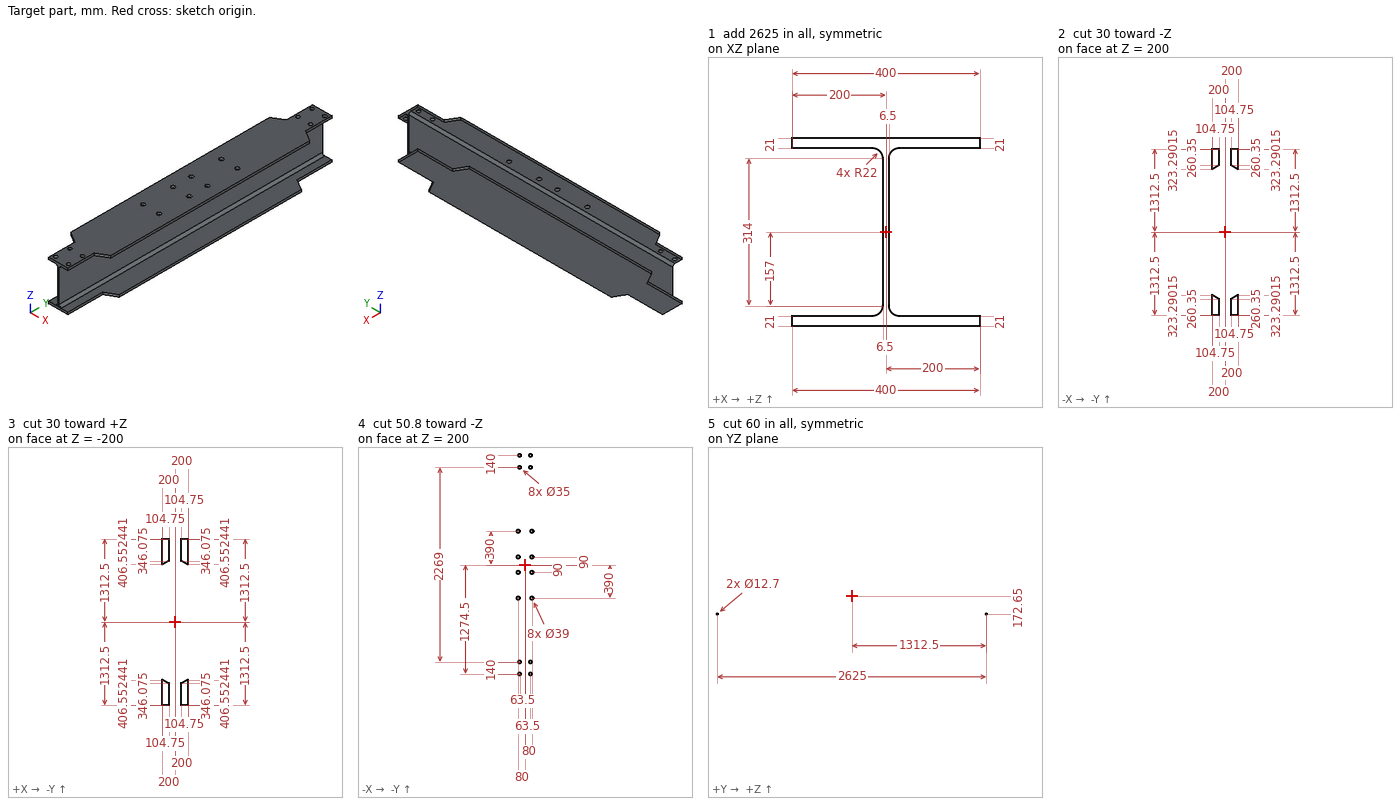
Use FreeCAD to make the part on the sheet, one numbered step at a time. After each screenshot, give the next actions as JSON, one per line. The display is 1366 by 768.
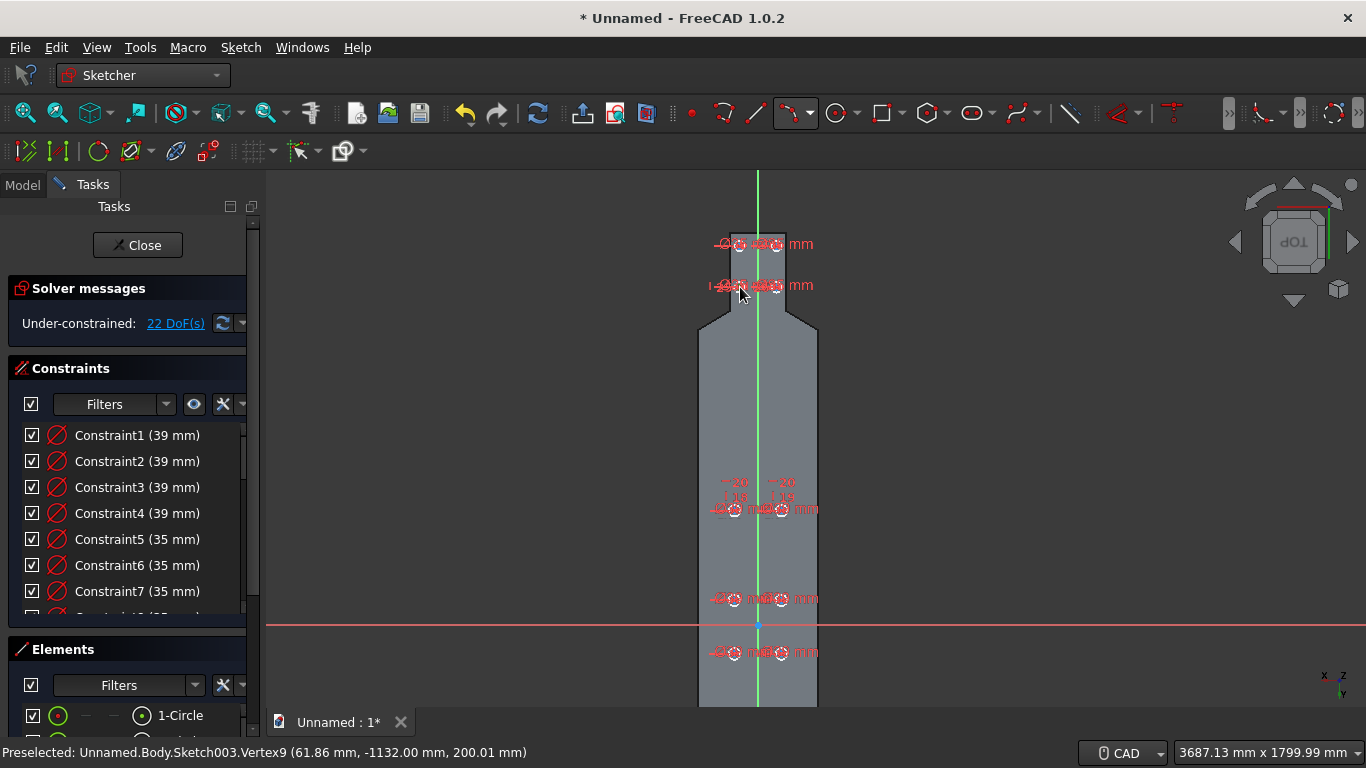
{"action": "left_click", "coordinate": [777, 287]}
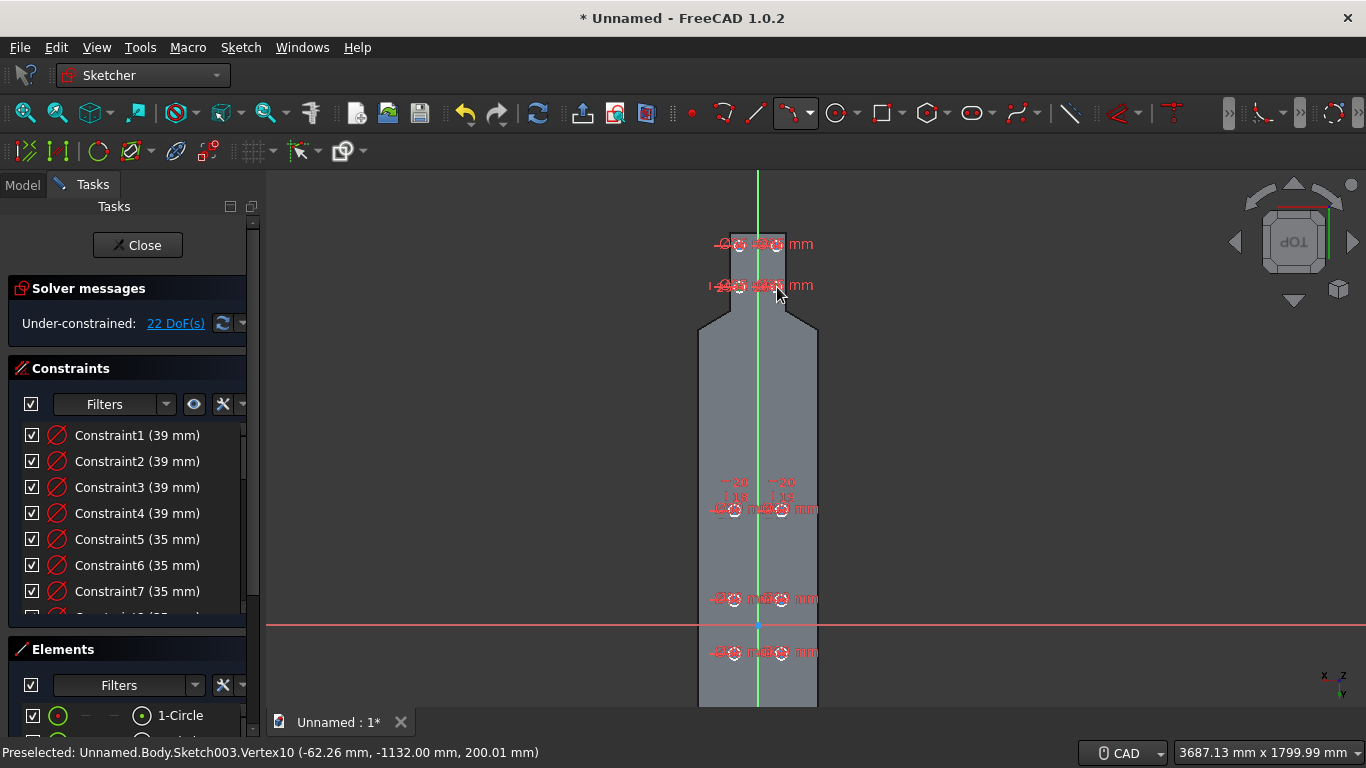
{"action": "key", "text": "h"}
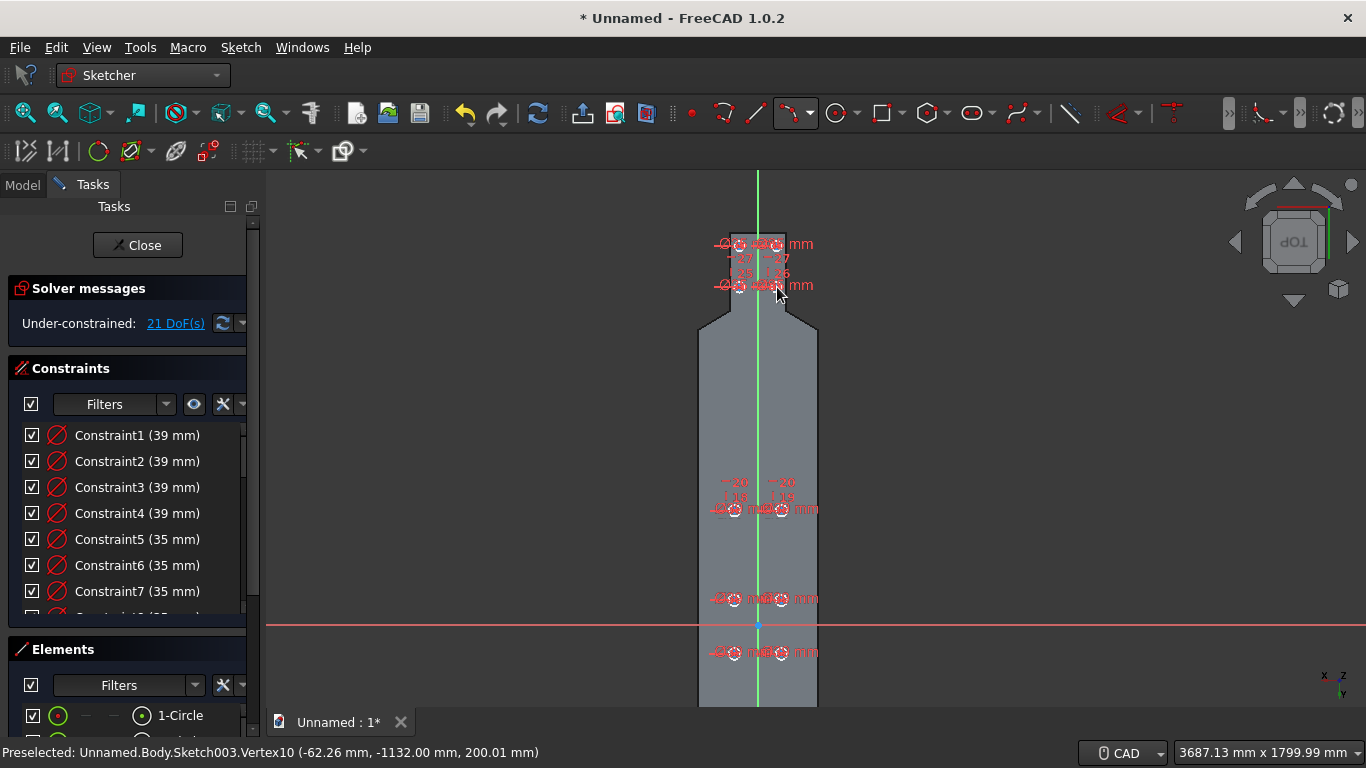
{"action": "left_click", "coordinate": [740, 287]}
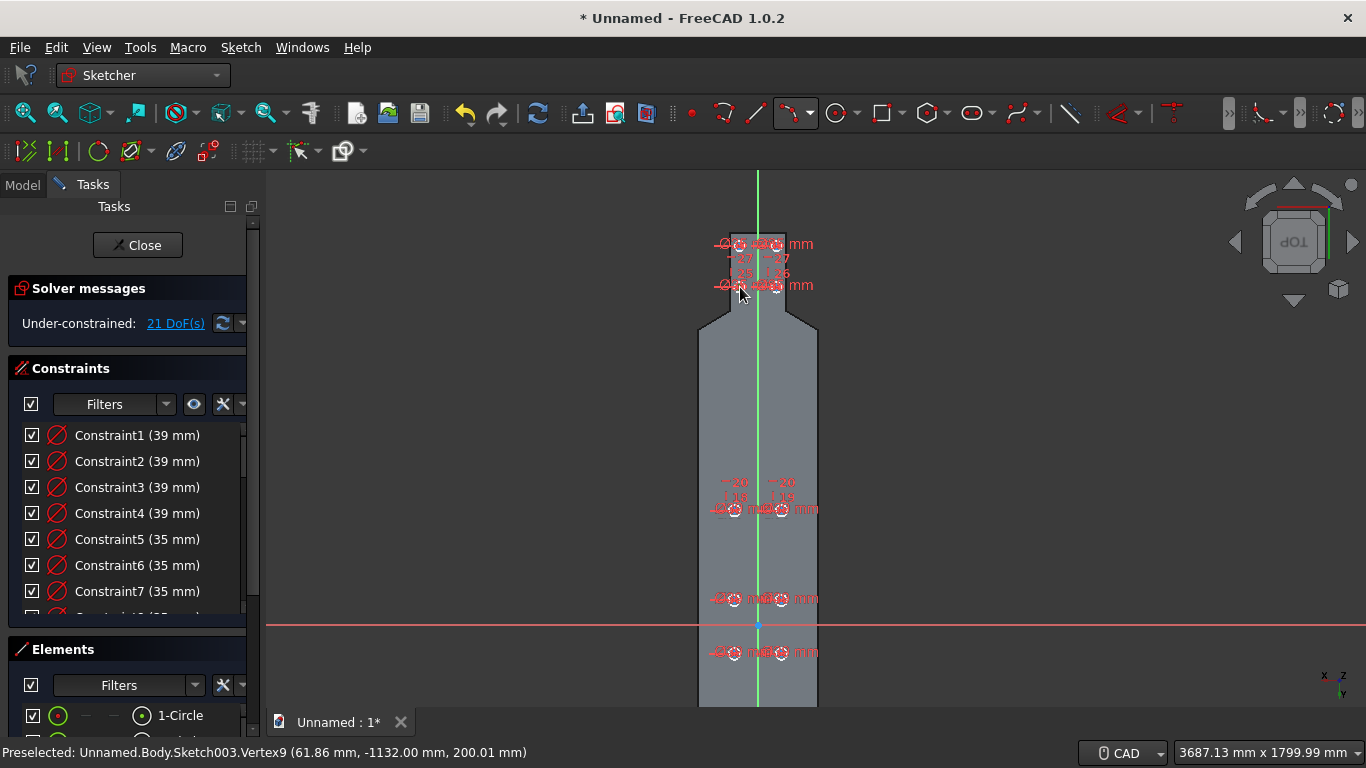
{"action": "left_click", "coordinate": [740, 246]}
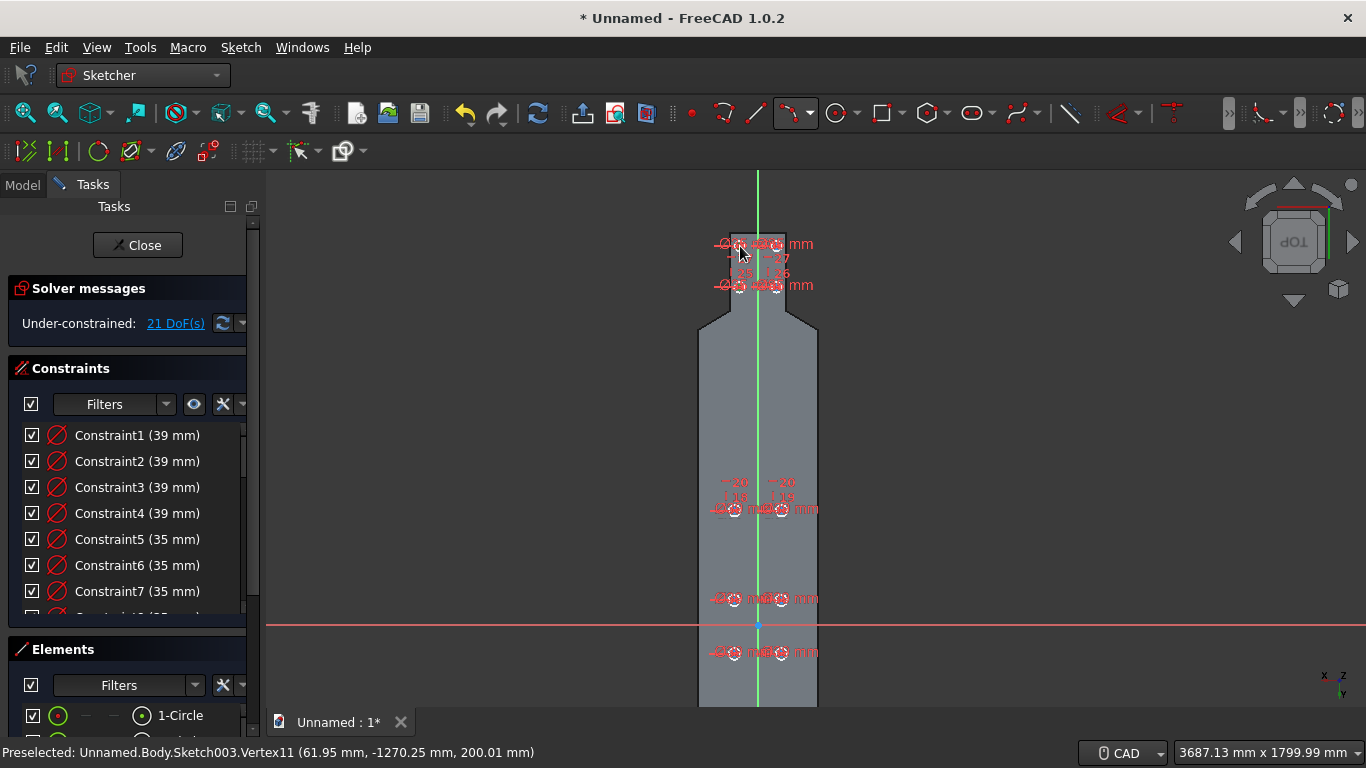
{"action": "key", "text": "v"}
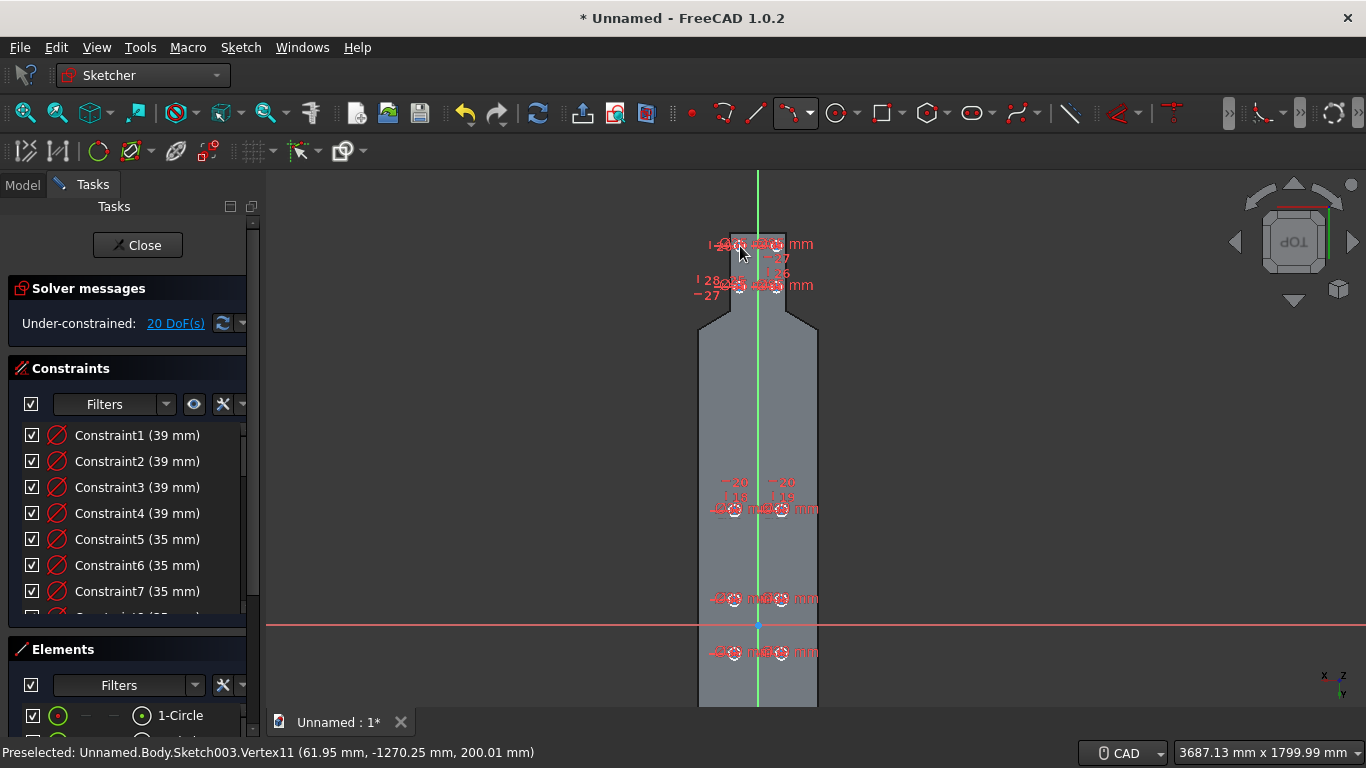
{"action": "left_click", "coordinate": [777, 287]}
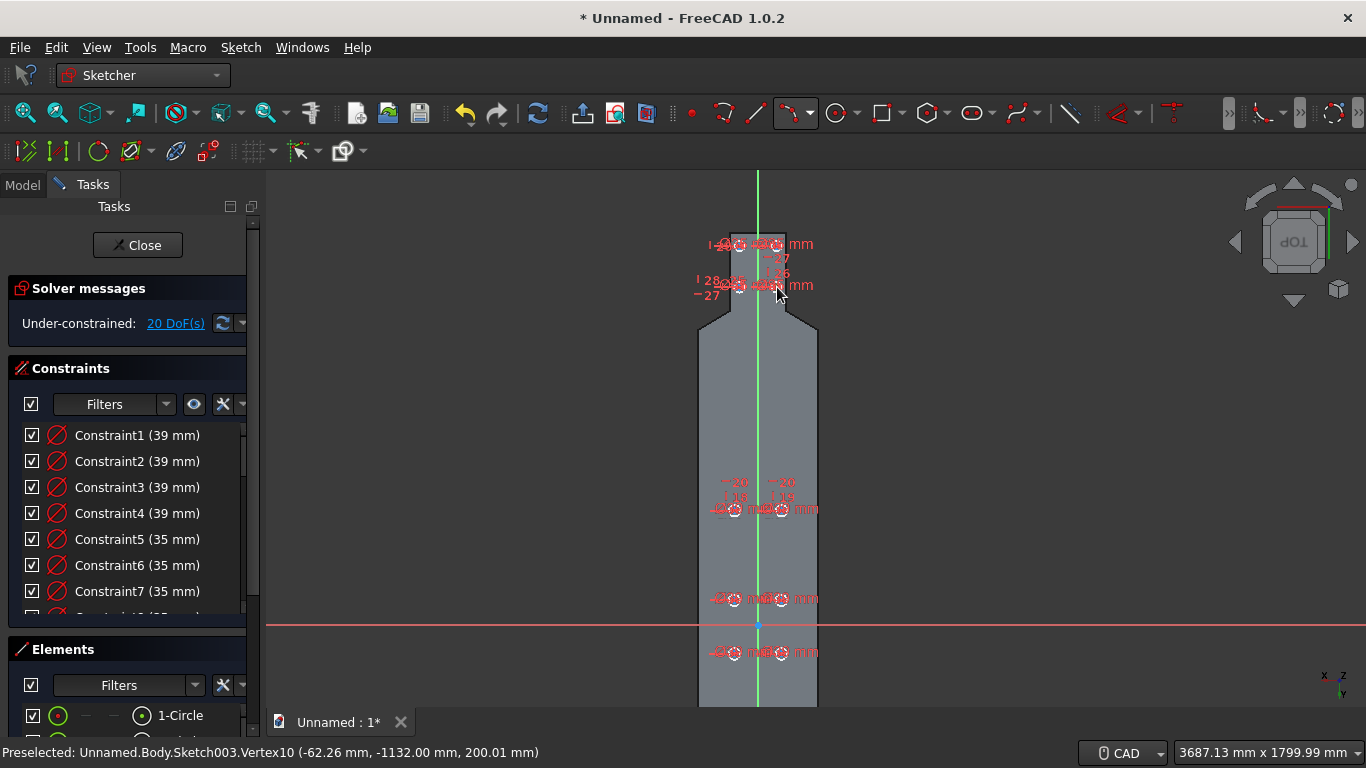
{"action": "left_click", "coordinate": [777, 246]}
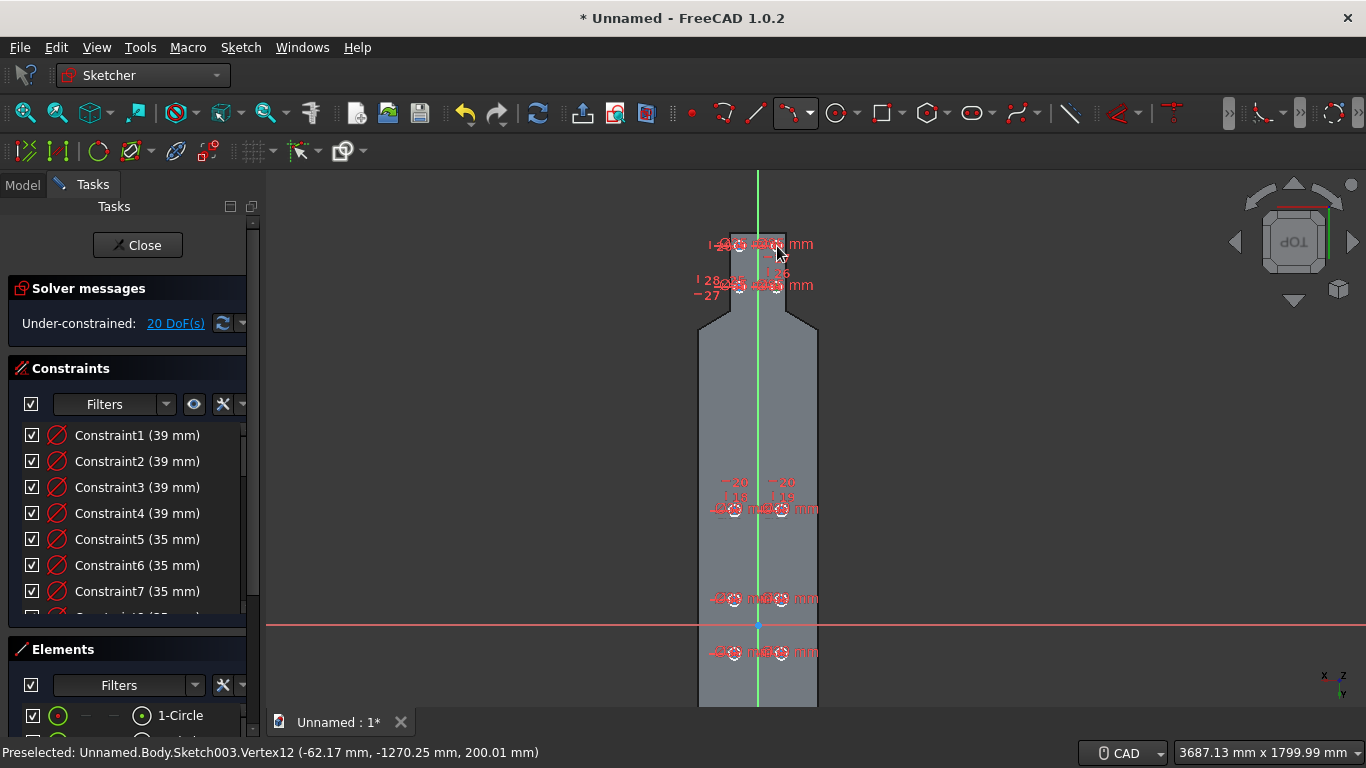
{"action": "key", "text": "v"}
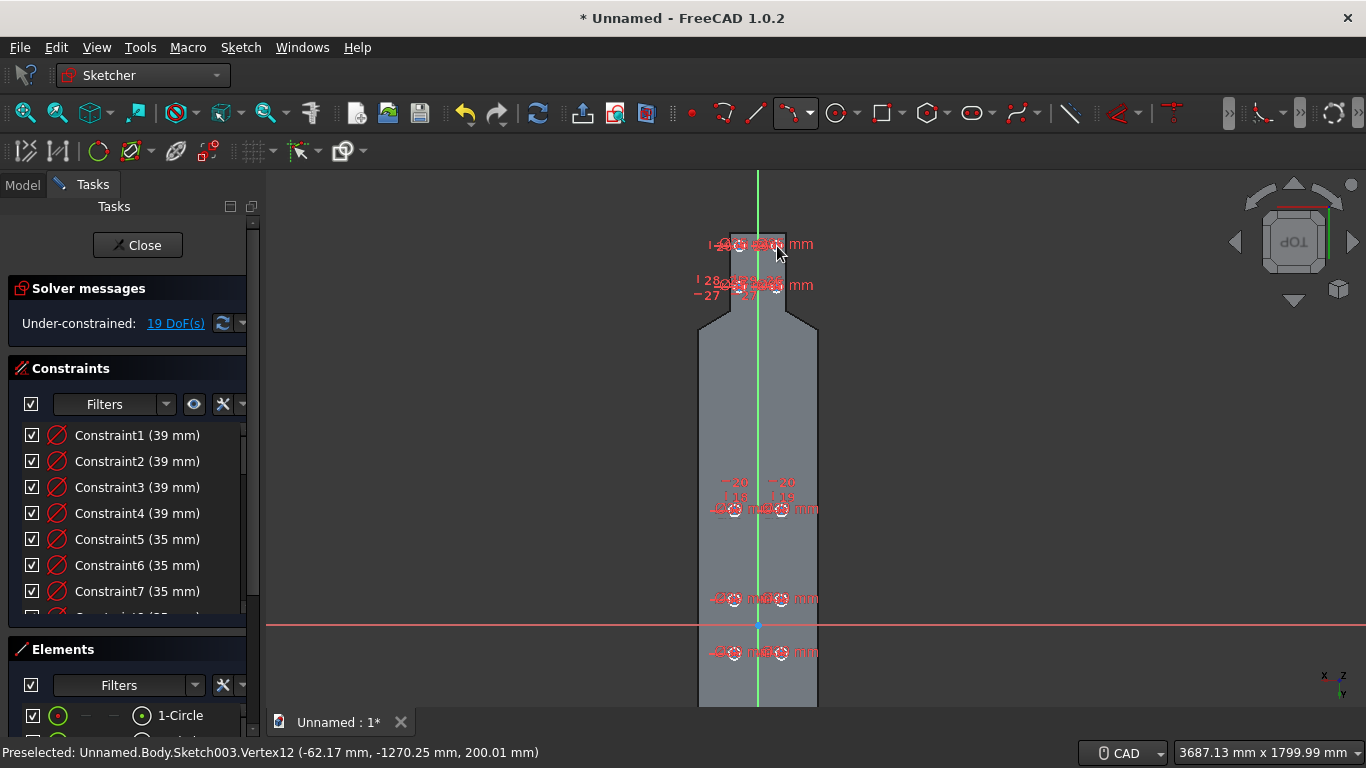
{"action": "left_click", "coordinate": [740, 246]}